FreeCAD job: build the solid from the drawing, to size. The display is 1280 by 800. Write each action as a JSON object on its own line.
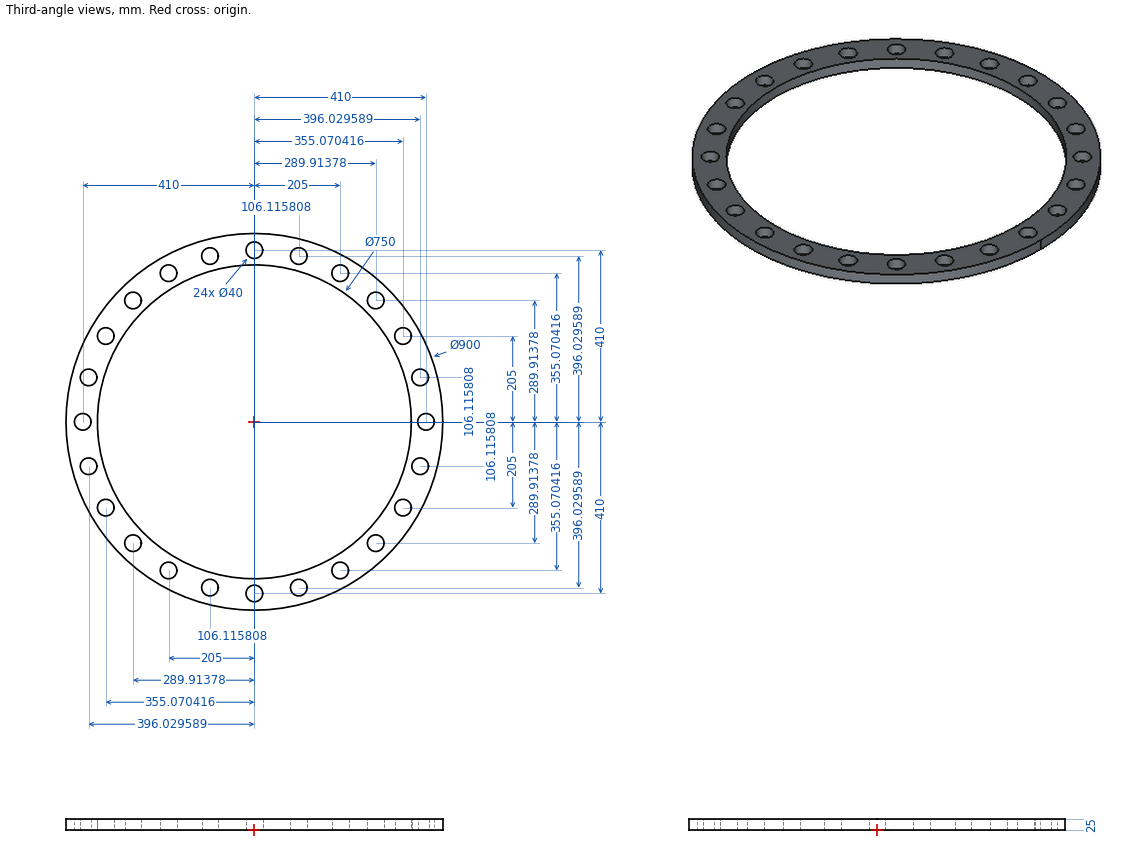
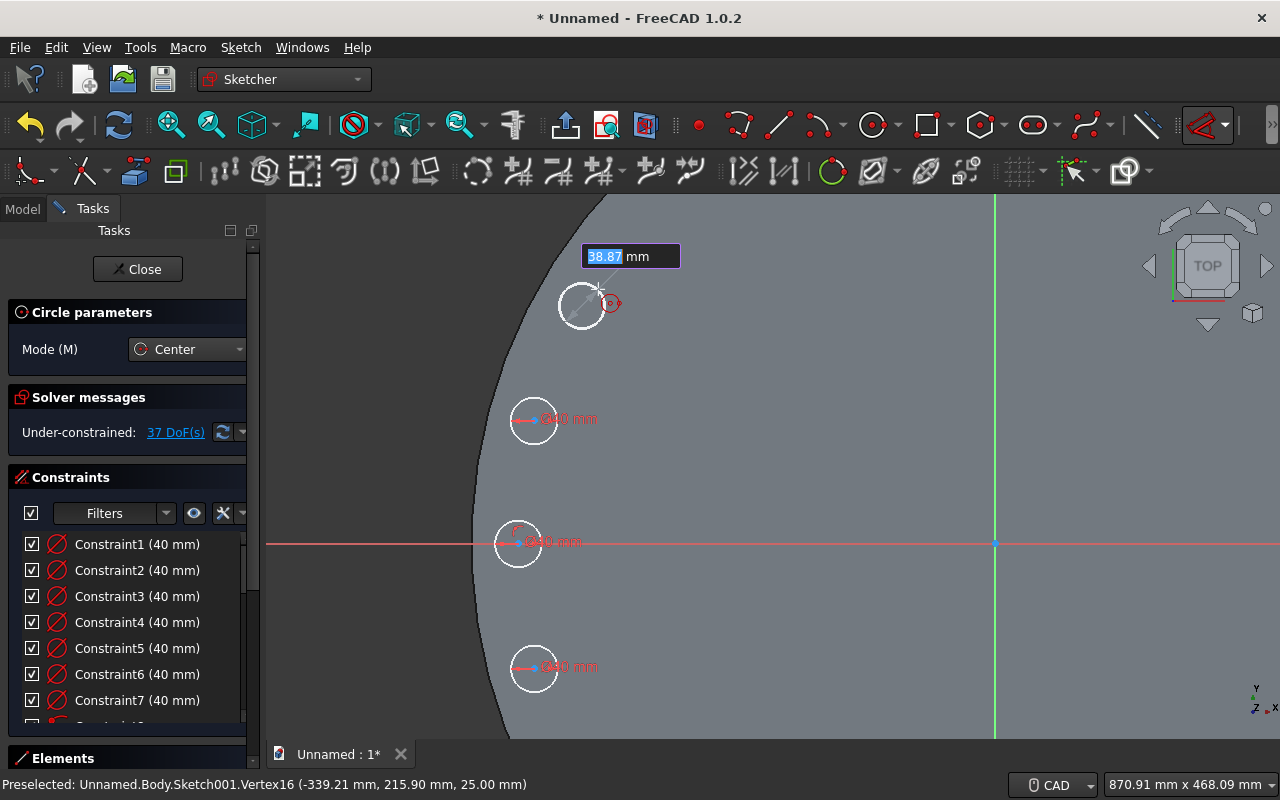
{"action": "type", "text": "40"}
{"action": "key", "text": "Return"}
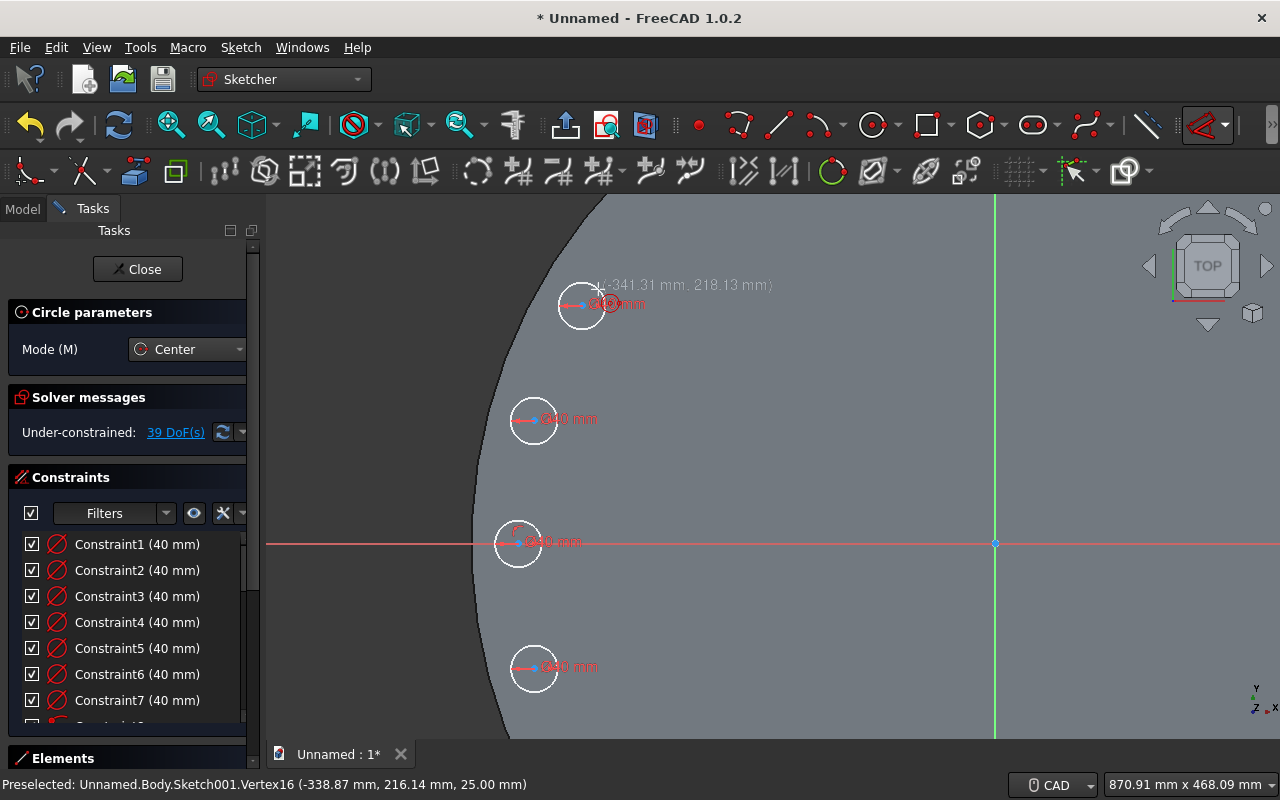
{"action": "scroll", "coordinate": [535, 421], "scroll_direction": "down", "scroll_amount": 5}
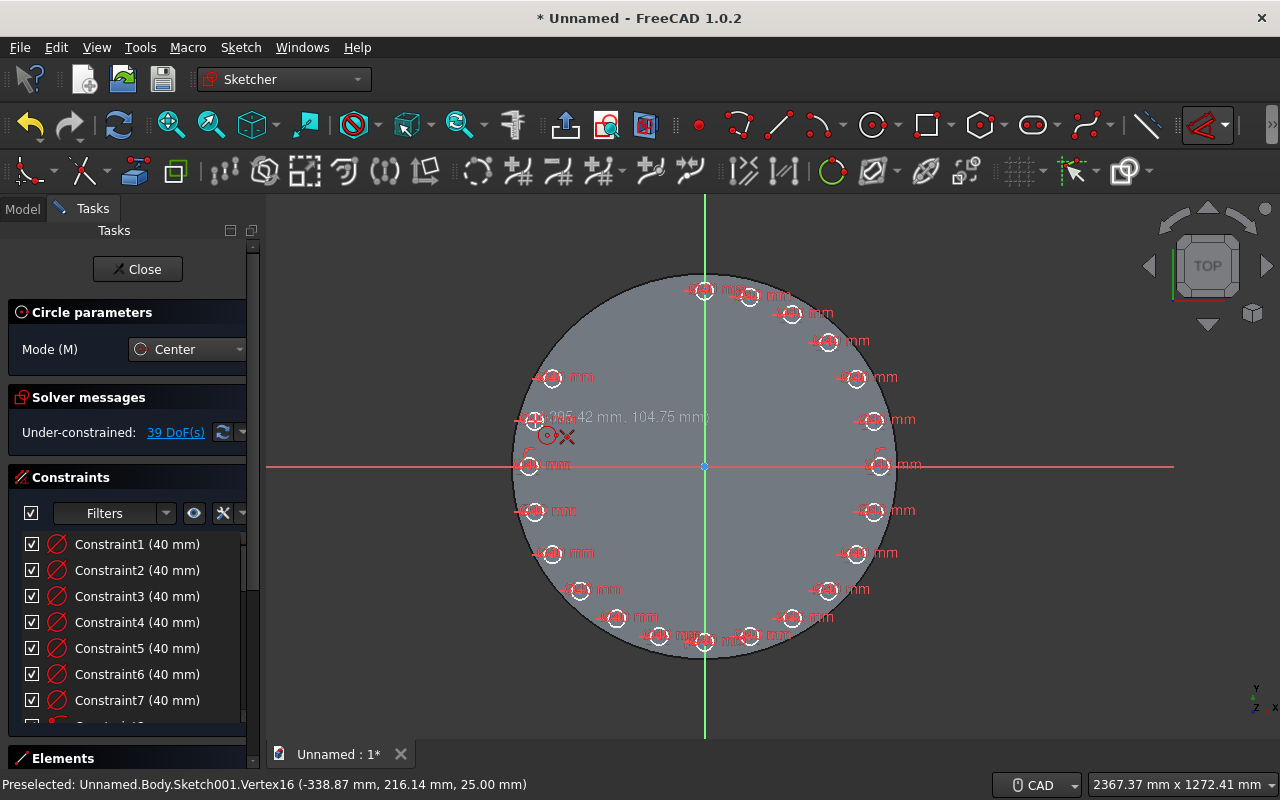
{"action": "scroll", "coordinate": [580, 342], "scroll_direction": "up", "scroll_amount": 5}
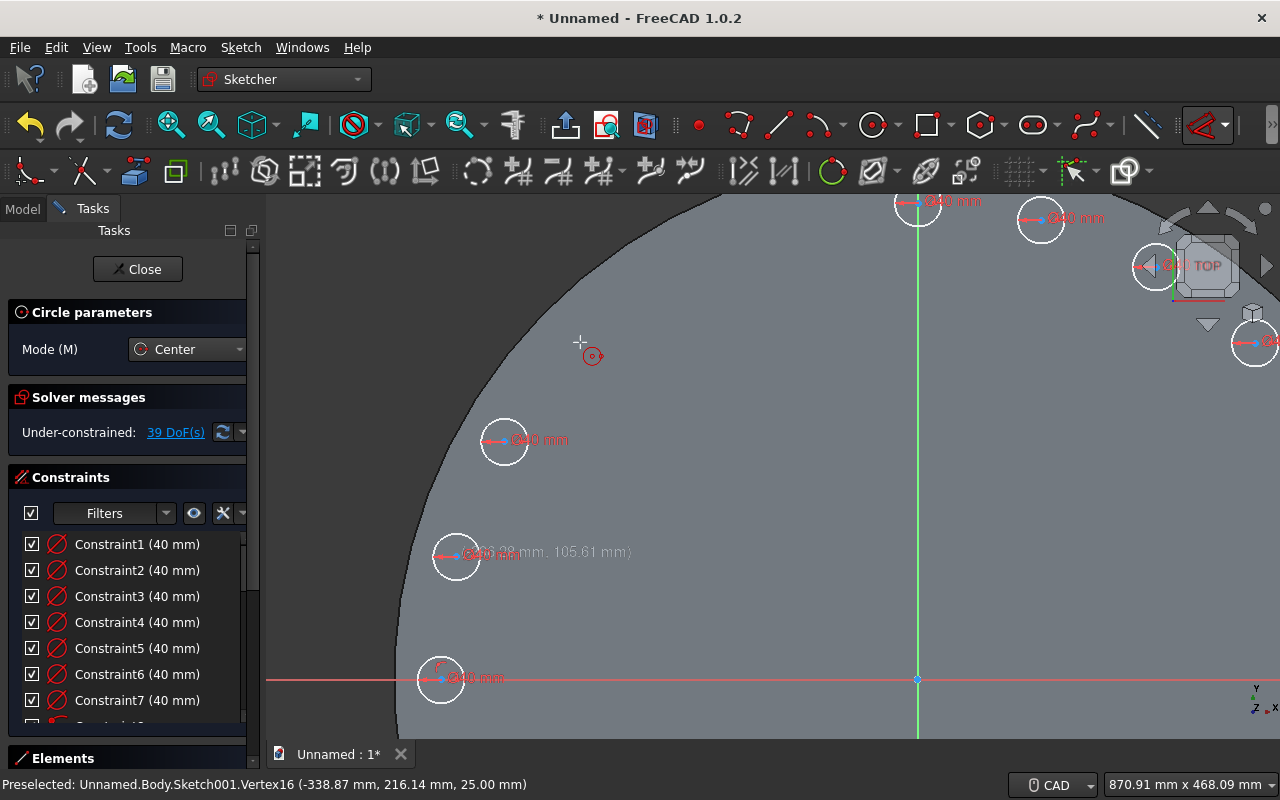
{"action": "left_click", "coordinate": [580, 342]}
{"action": "mouse_move", "coordinate": [597, 326]}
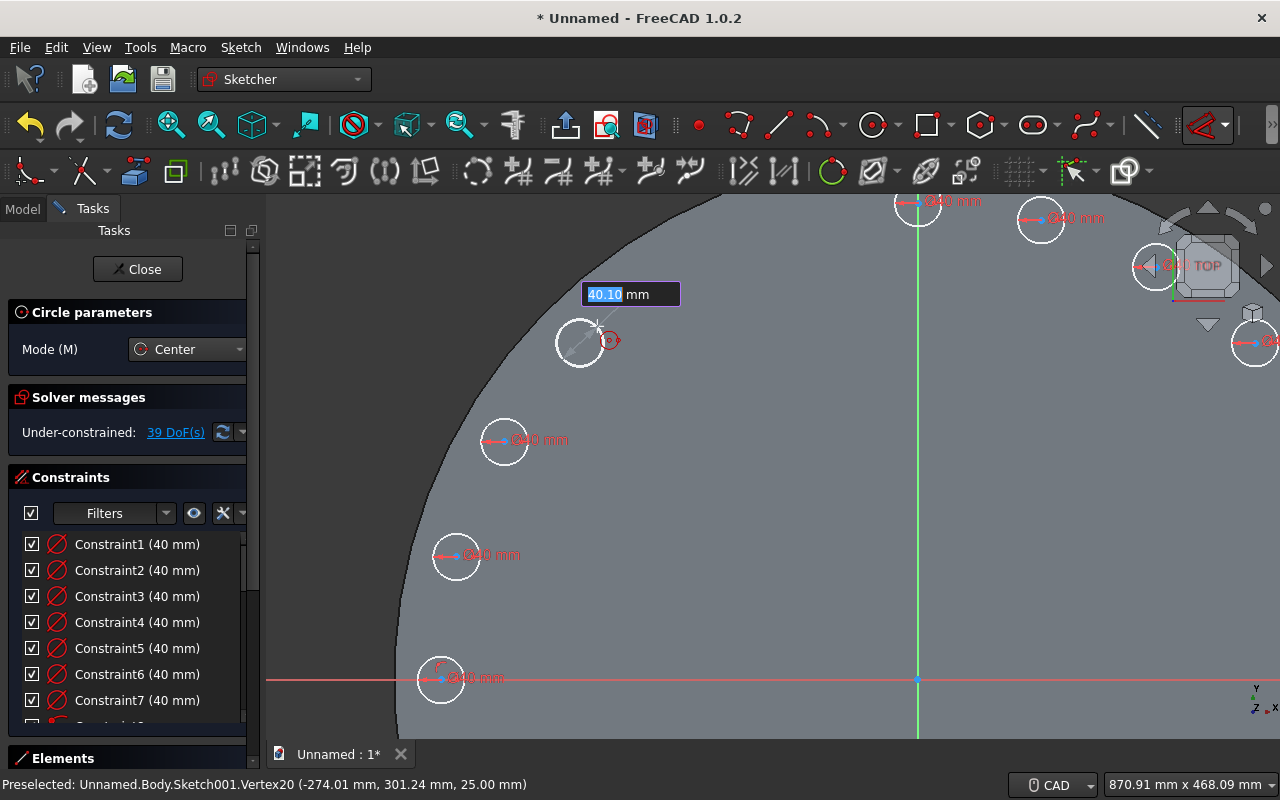
{"action": "type", "text": "40"}
{"action": "key", "text": "Return"}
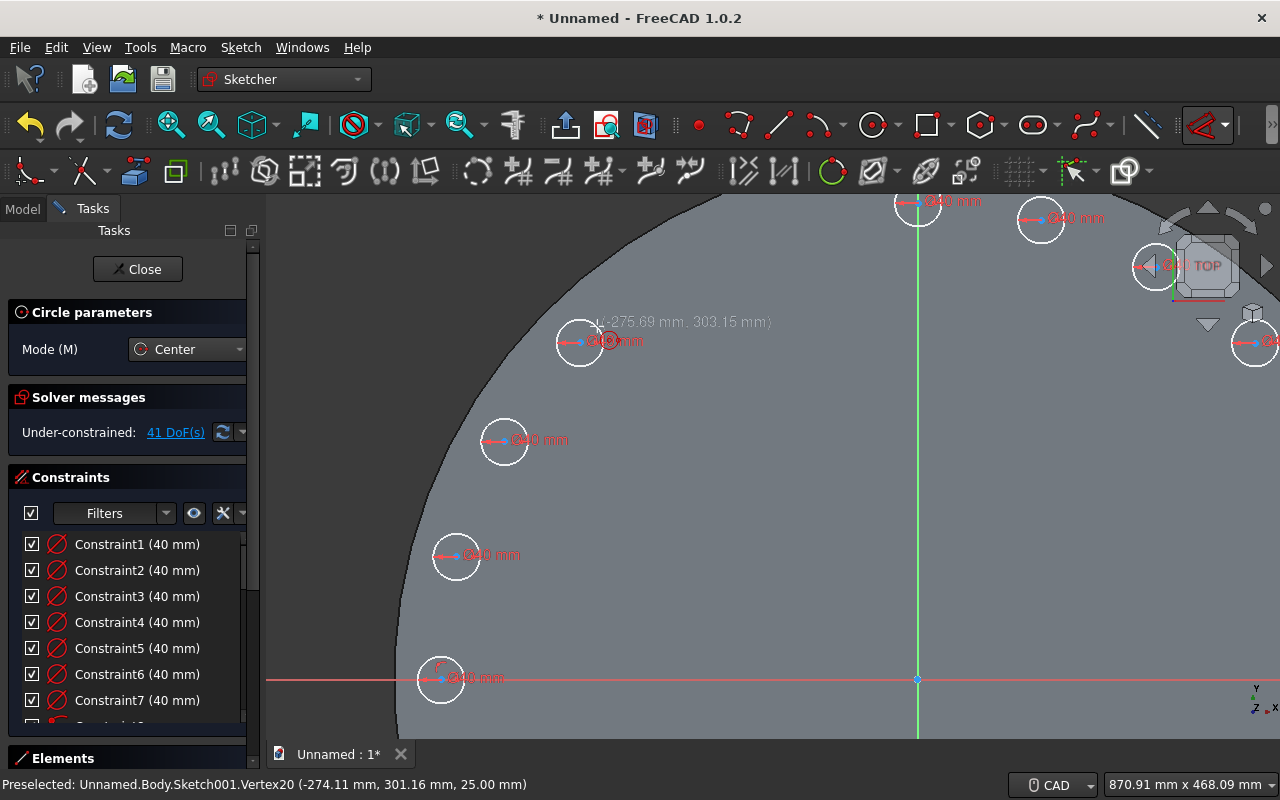
{"action": "left_click", "coordinate": [679, 267]}
{"action": "mouse_move", "coordinate": [696, 250]}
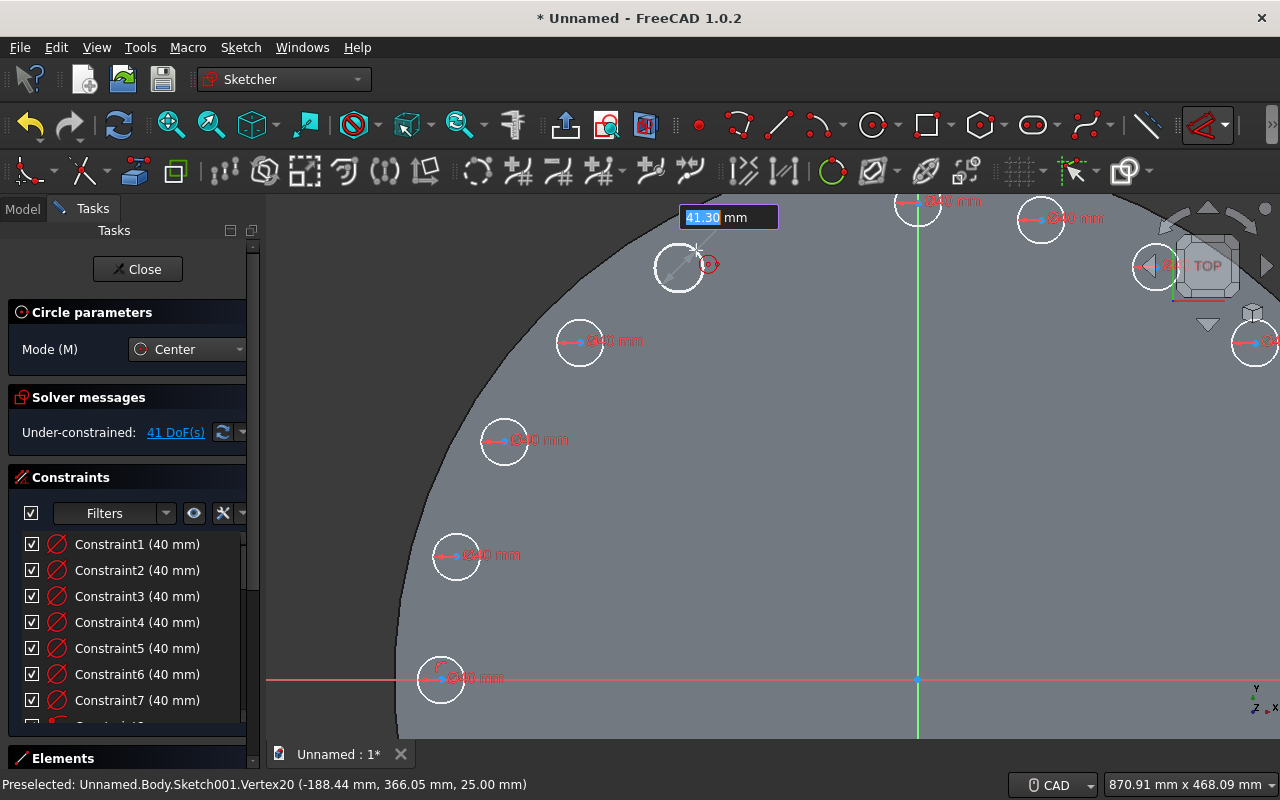
{"action": "type", "text": "40"}
{"action": "key", "text": "Return"}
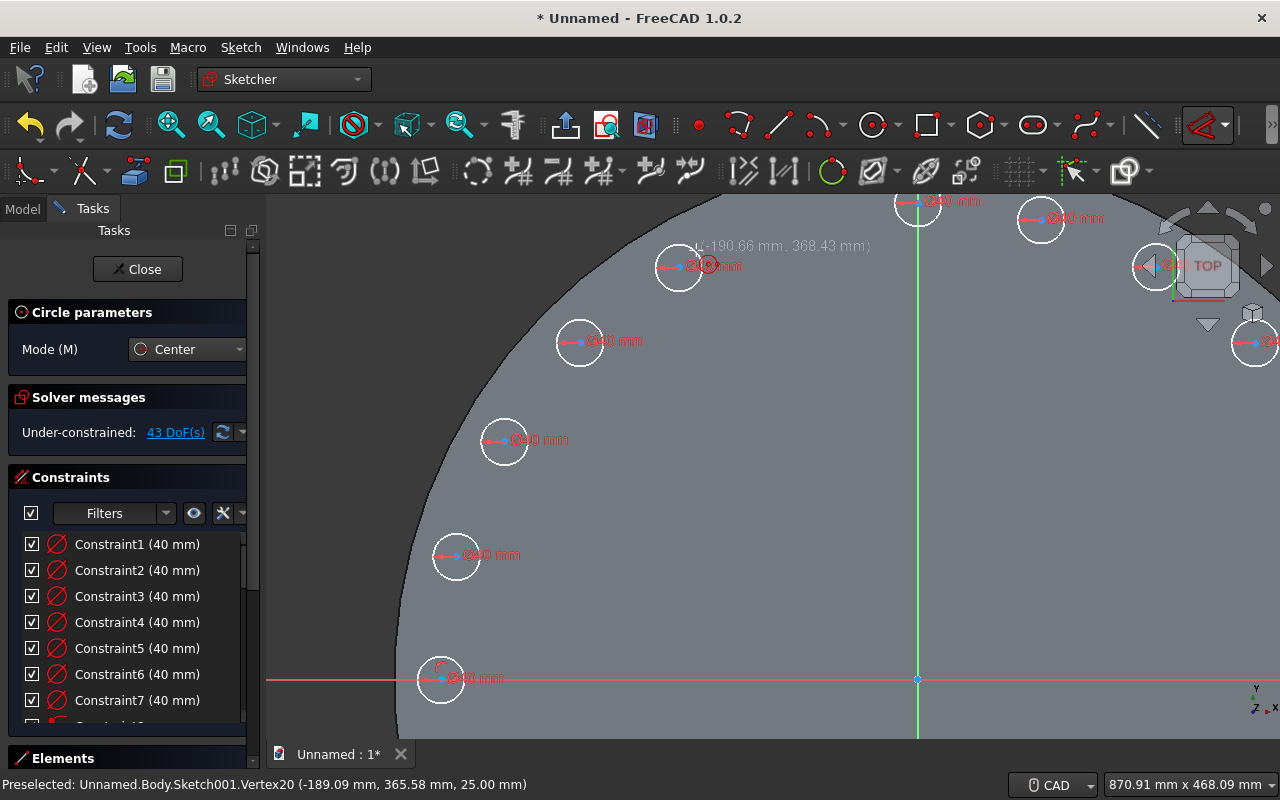
{"action": "scroll", "coordinate": [580, 342], "scroll_direction": "down", "scroll_amount": 5}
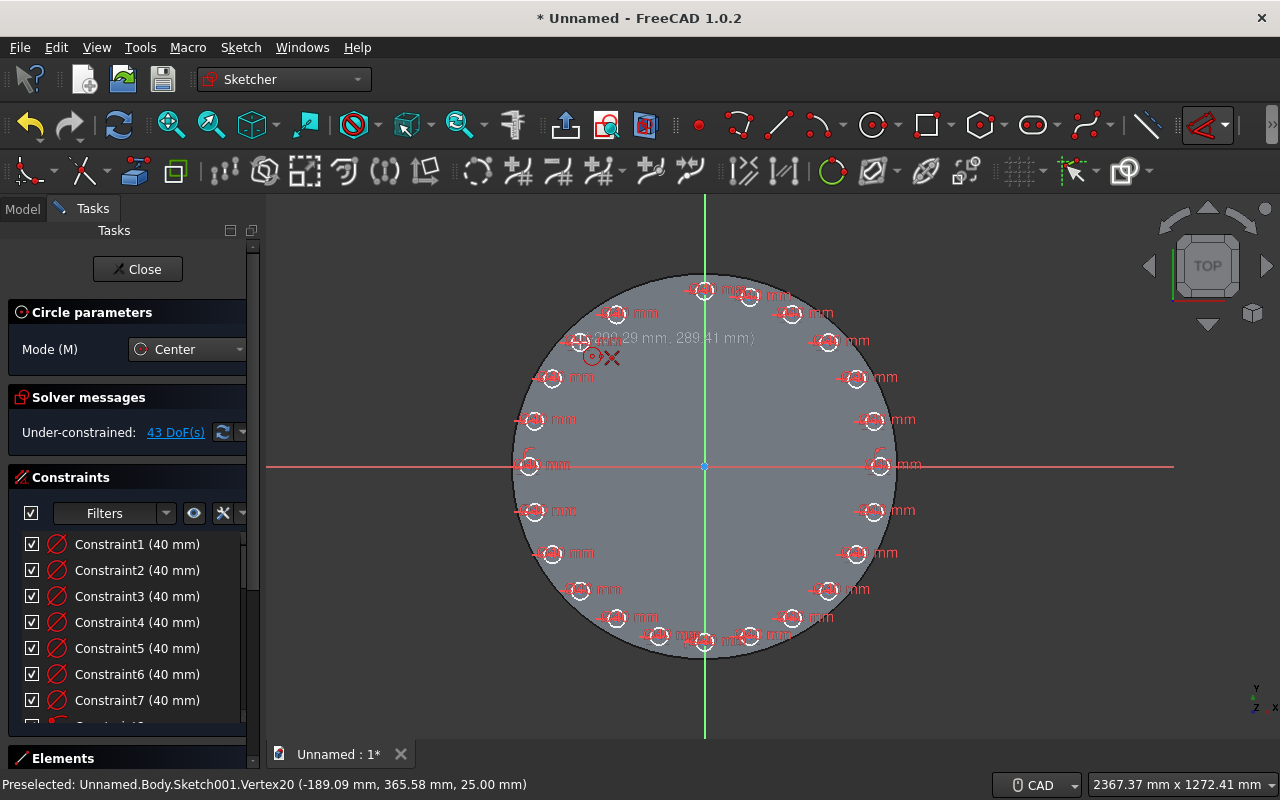
{"action": "scroll", "coordinate": [659, 297], "scroll_direction": "up", "scroll_amount": 5}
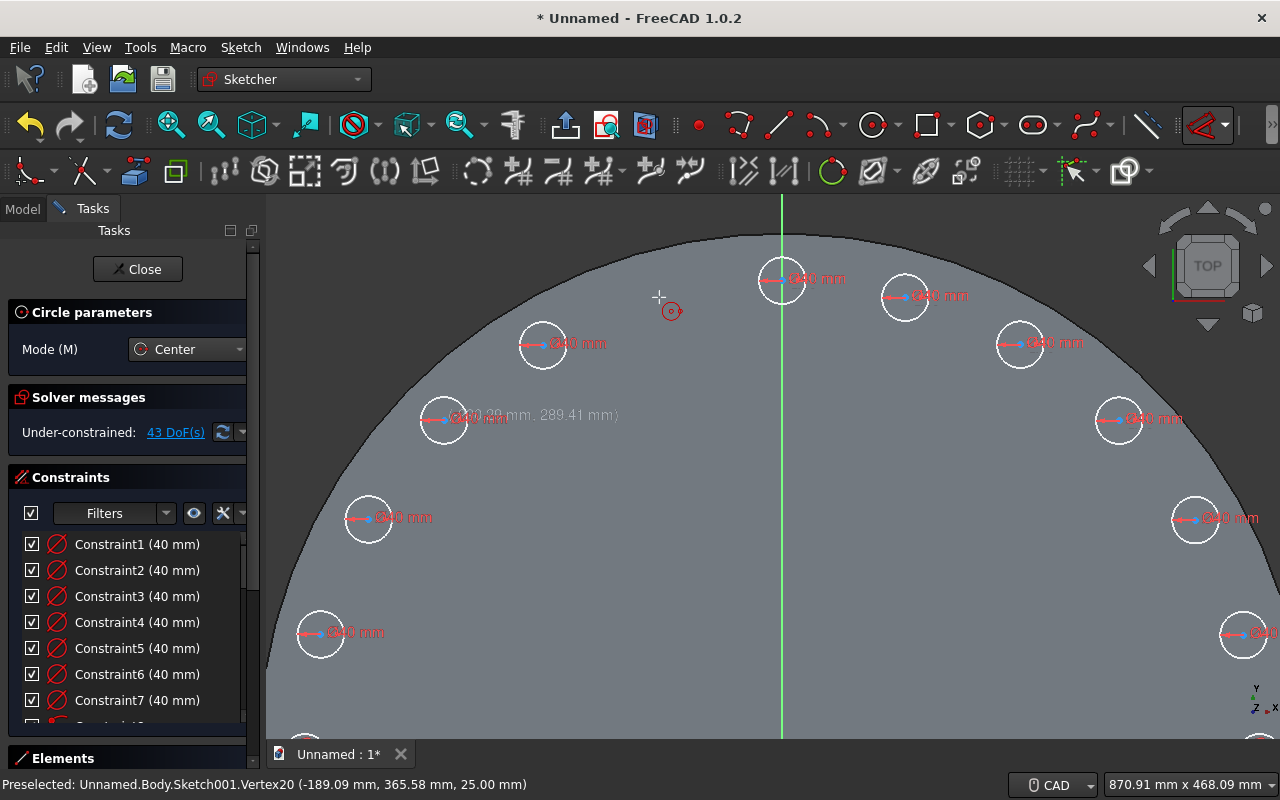
{"action": "left_click", "coordinate": [659, 296]}
{"action": "mouse_move", "coordinate": [675, 280]}